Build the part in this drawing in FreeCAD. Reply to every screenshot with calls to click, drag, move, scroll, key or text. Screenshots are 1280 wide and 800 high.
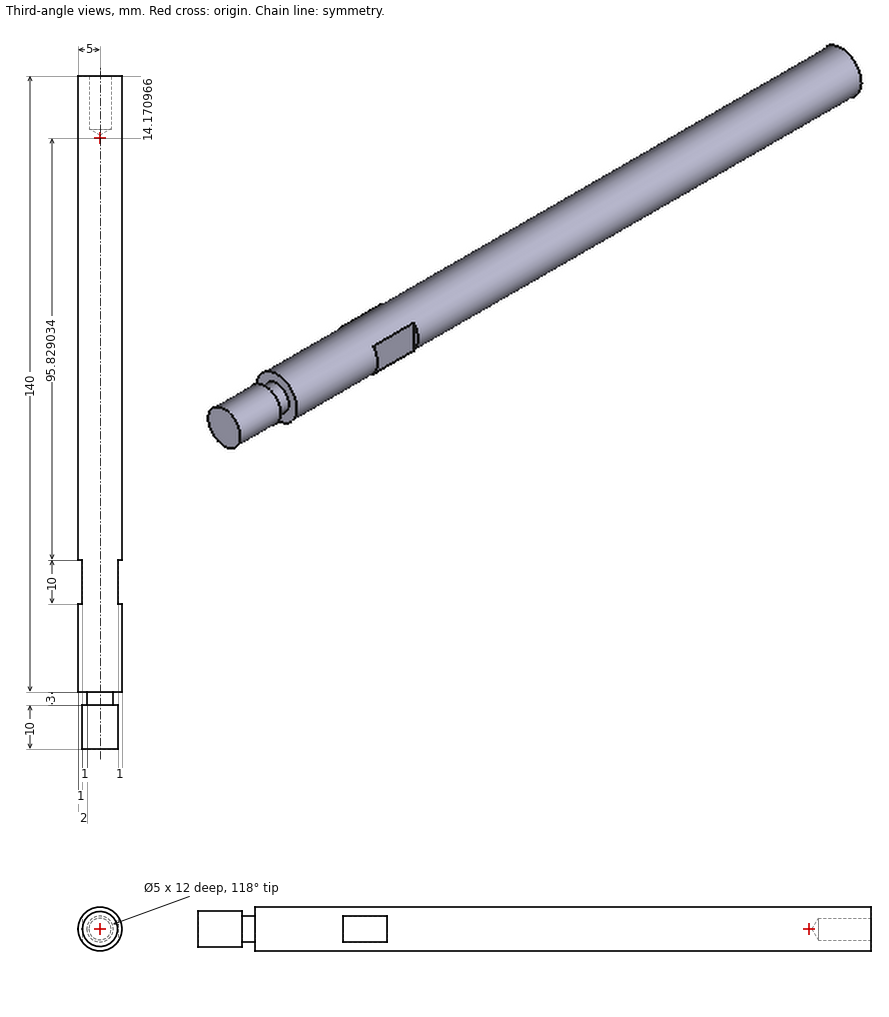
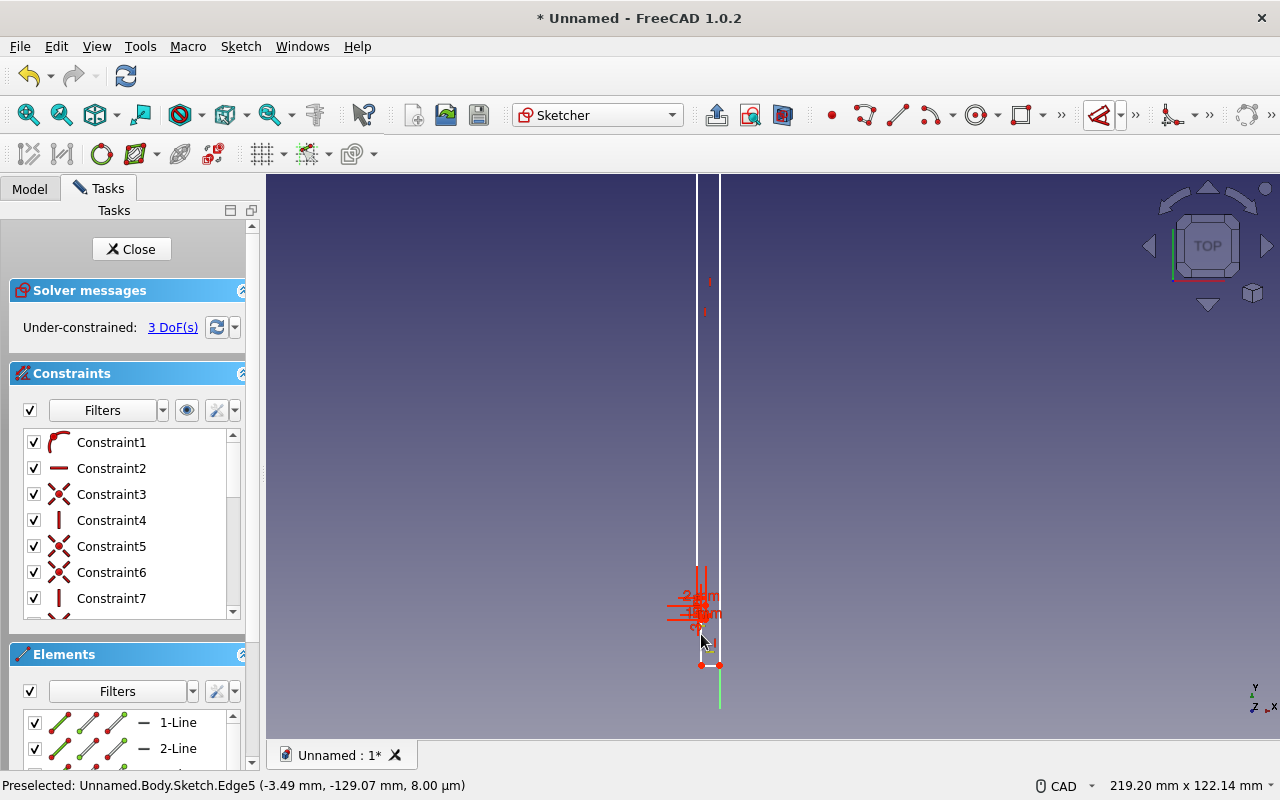
click(701, 652)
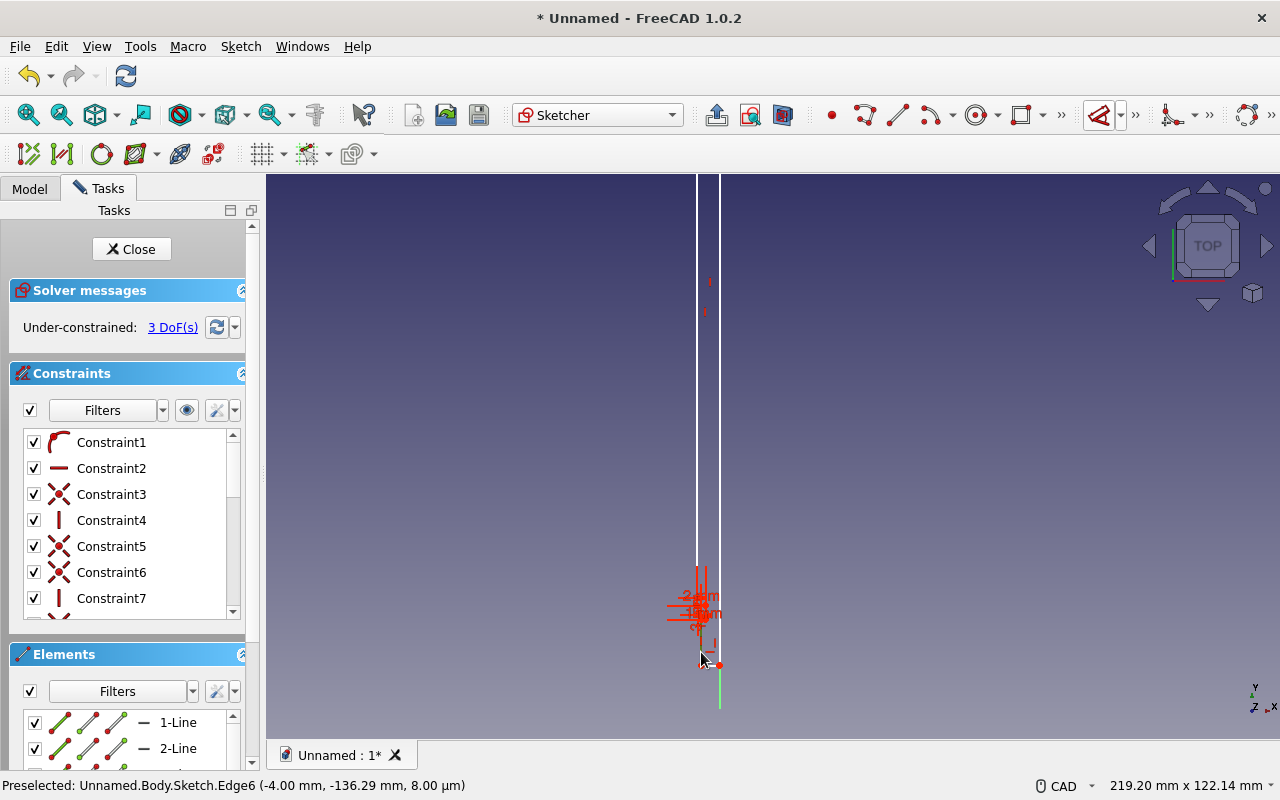
key(i)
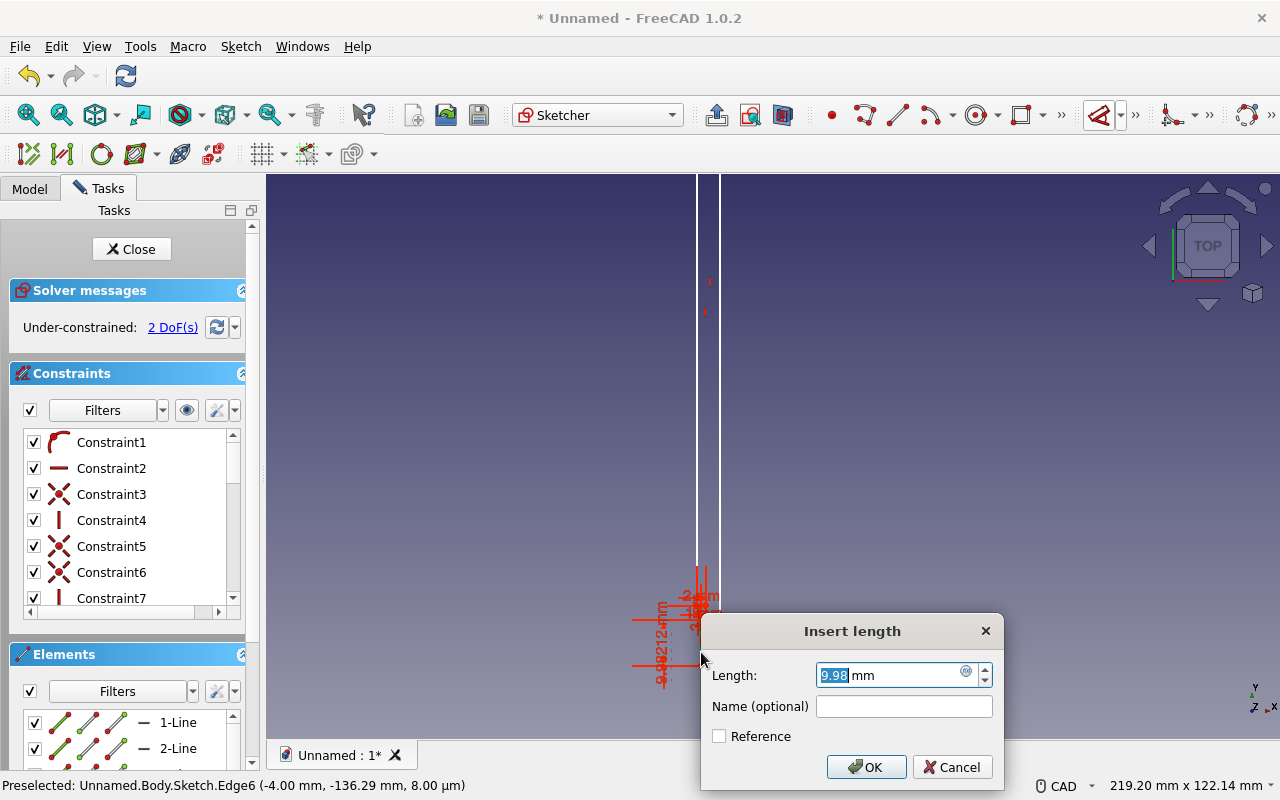
text(10)
key(Return)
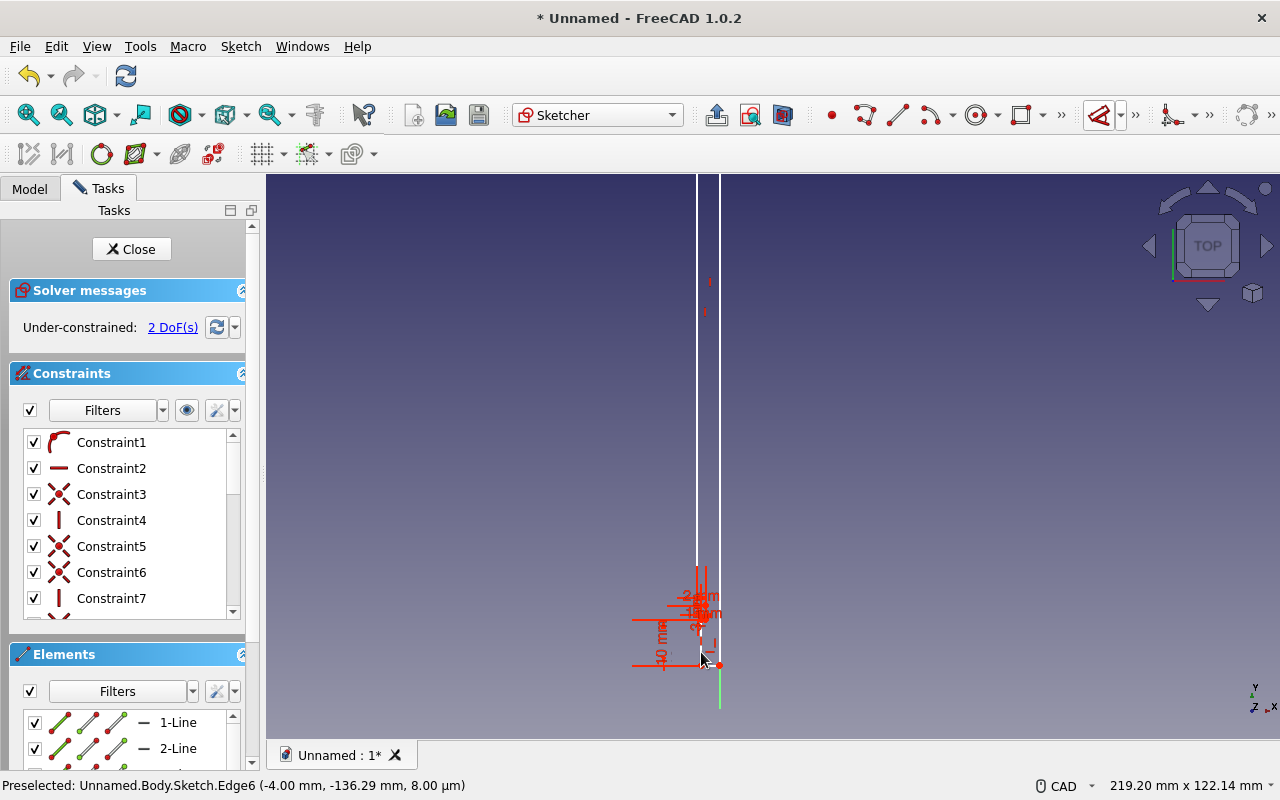
click(697, 411)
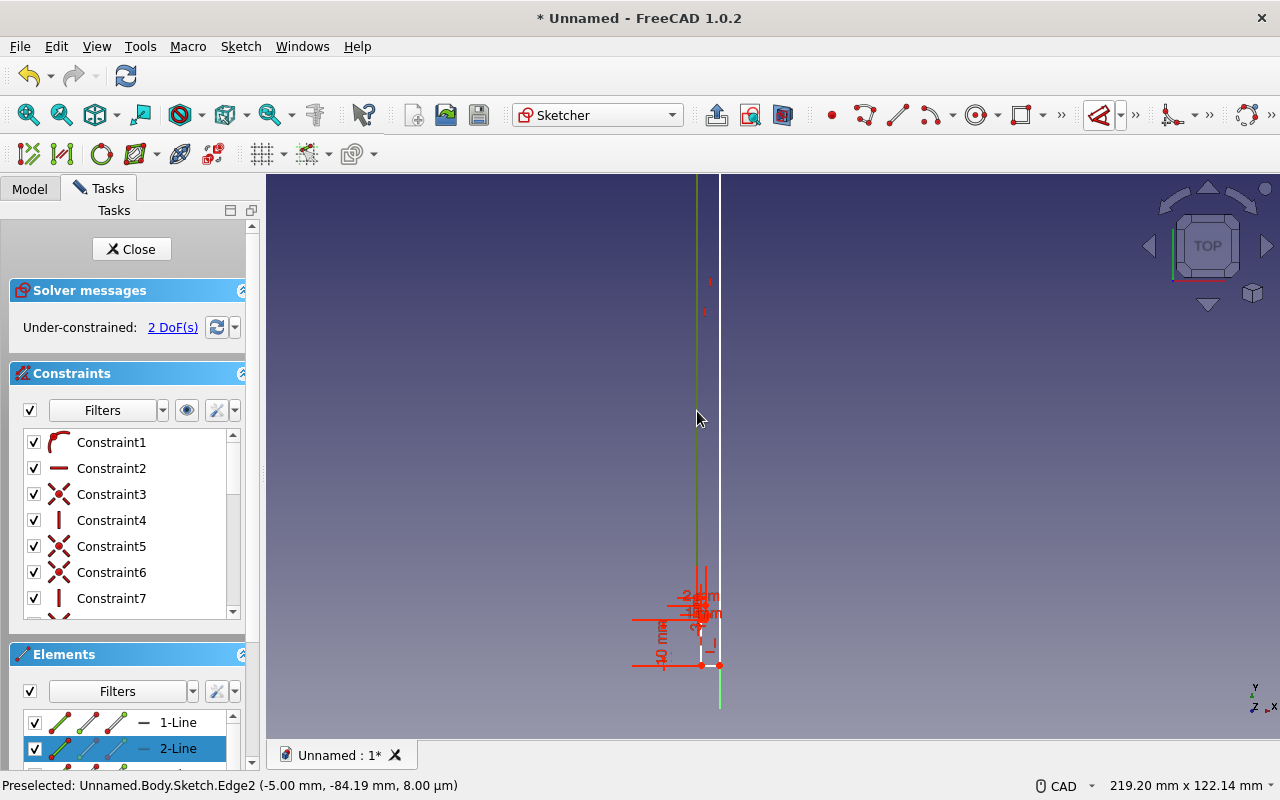
click(1120, 116)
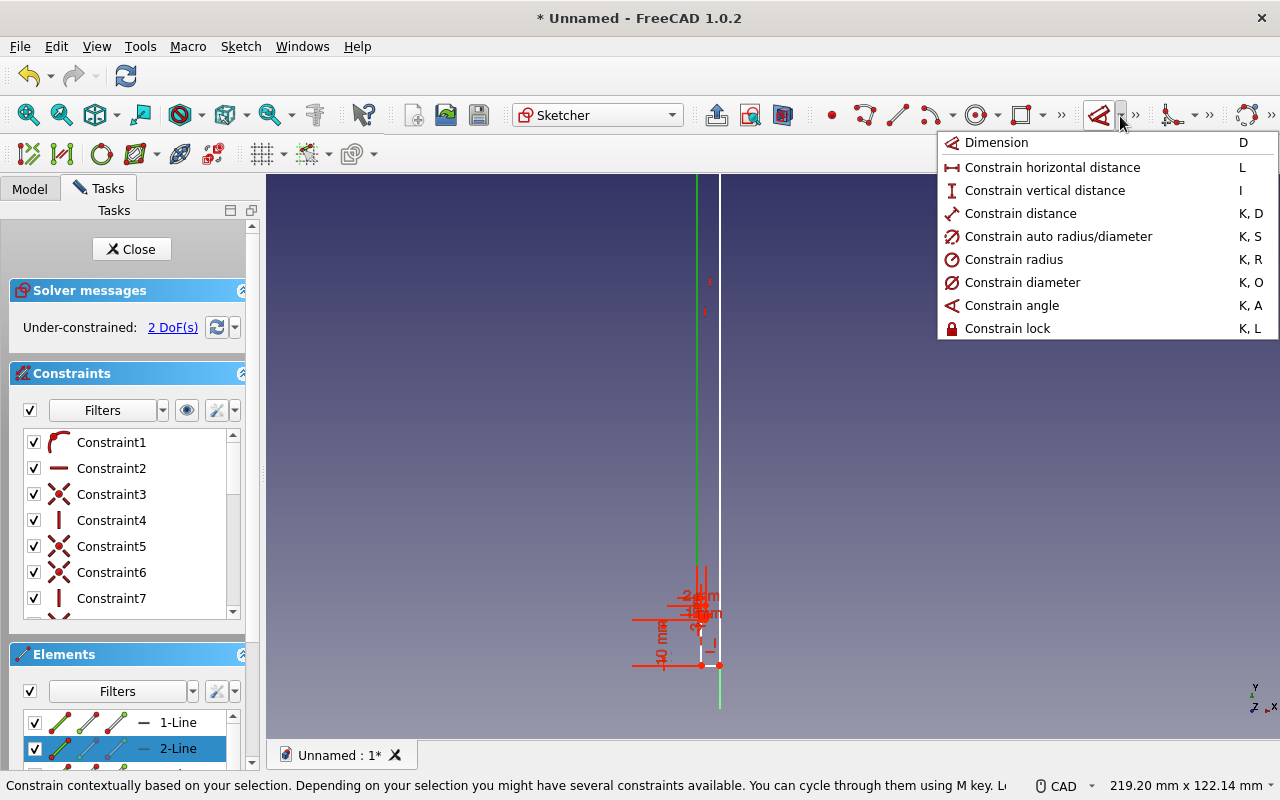
click(1108, 190)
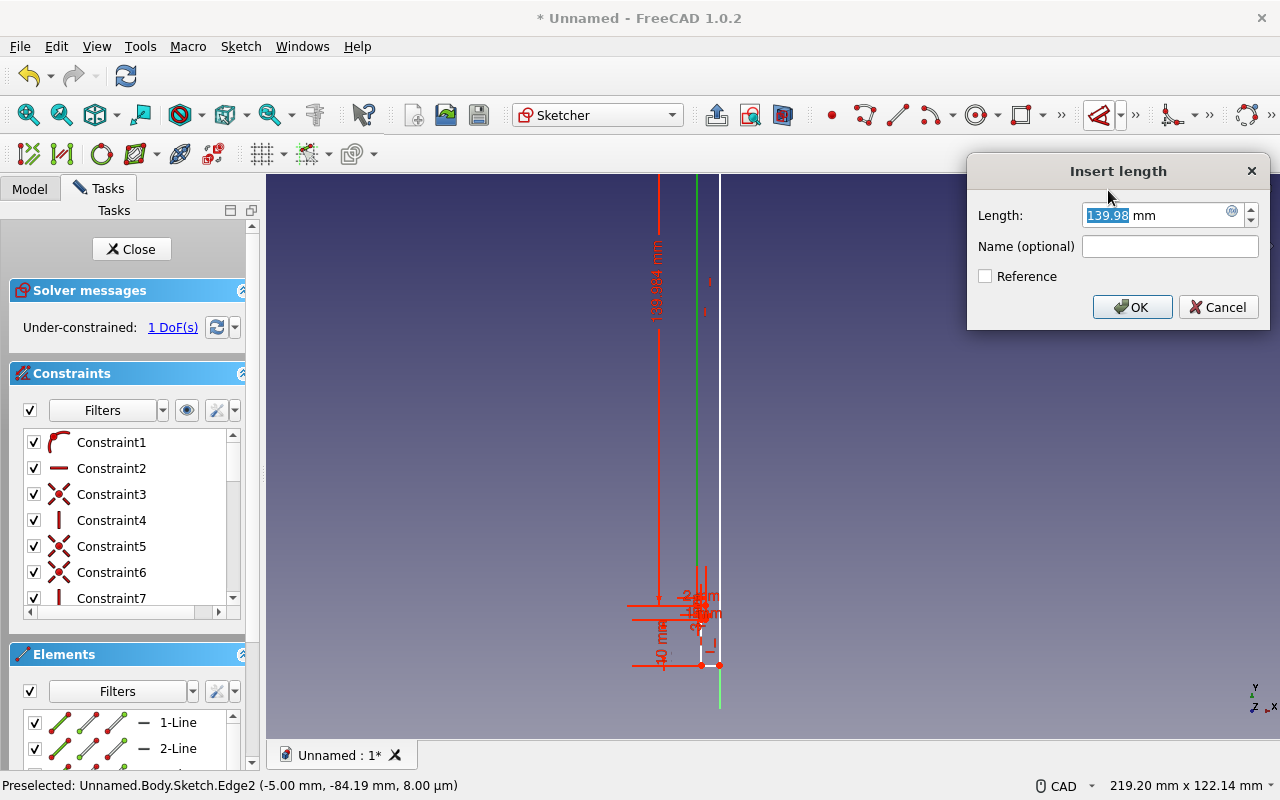
text(140)
key(Return)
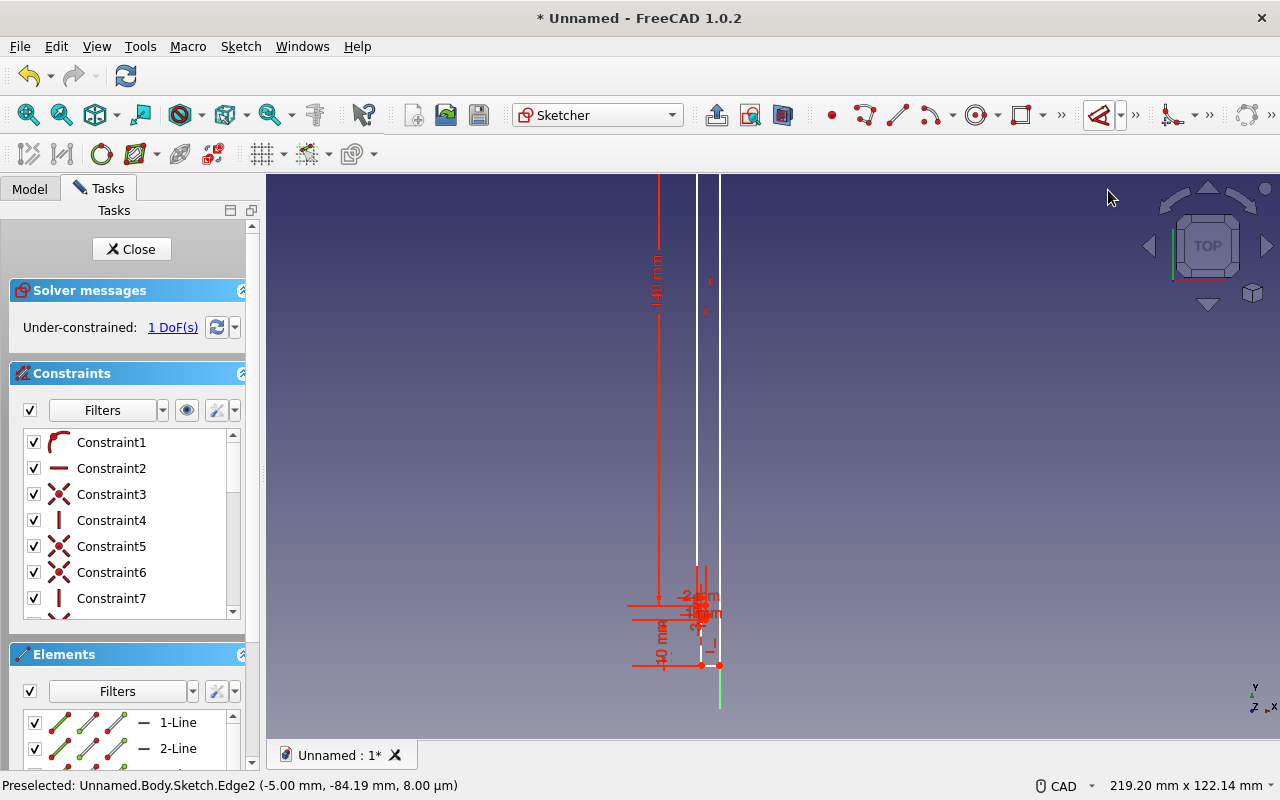
scroll(700, 634, down, 3)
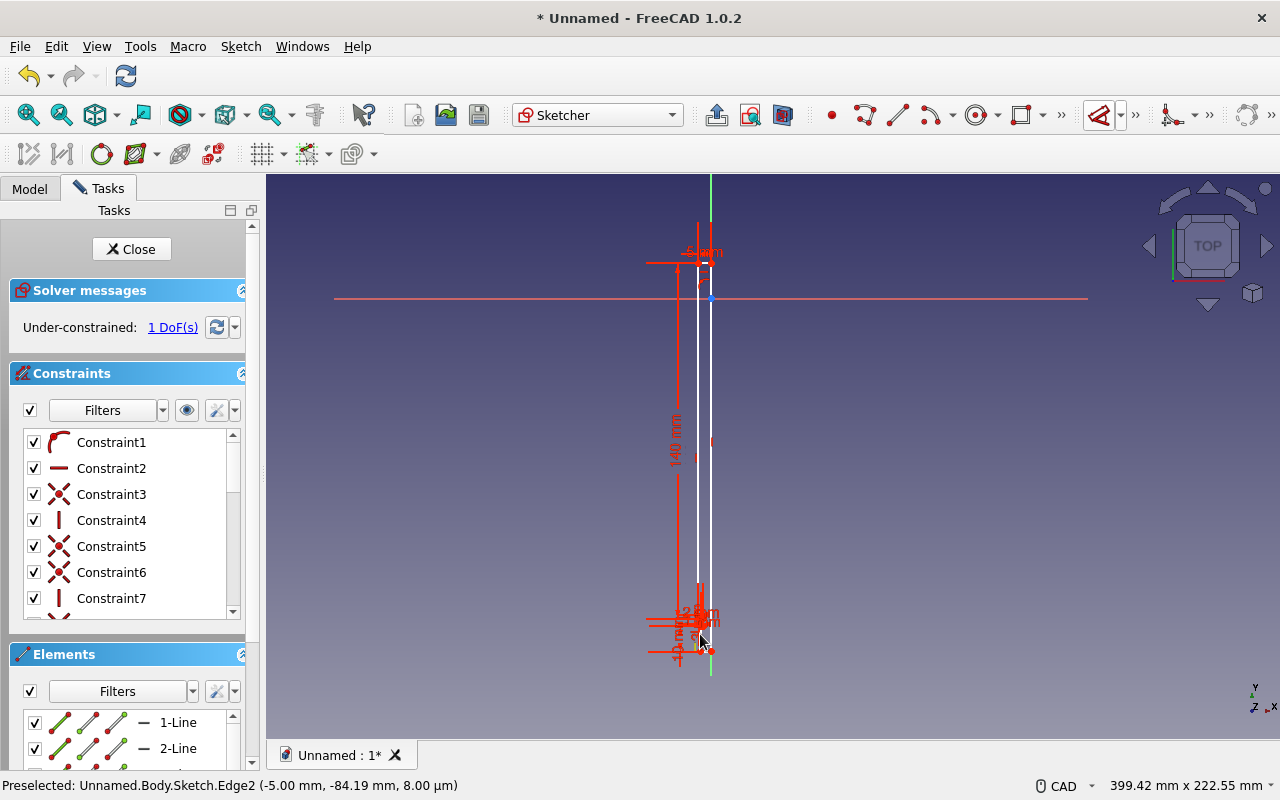
click(711, 263)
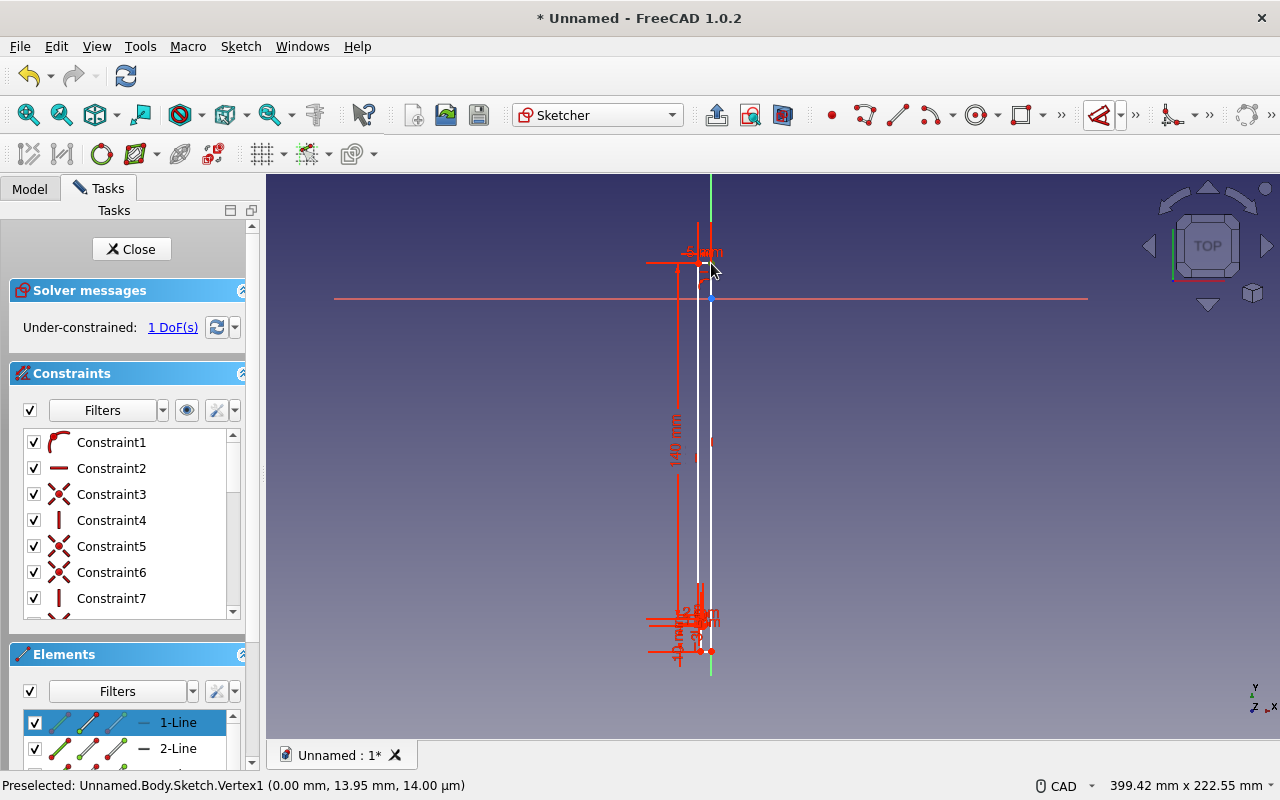
click(1120, 116)